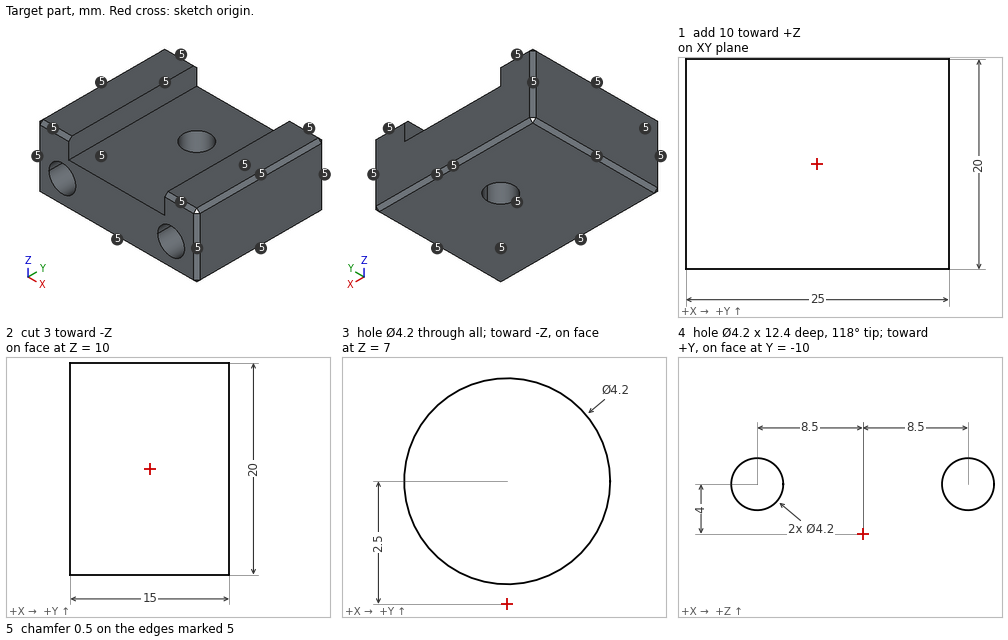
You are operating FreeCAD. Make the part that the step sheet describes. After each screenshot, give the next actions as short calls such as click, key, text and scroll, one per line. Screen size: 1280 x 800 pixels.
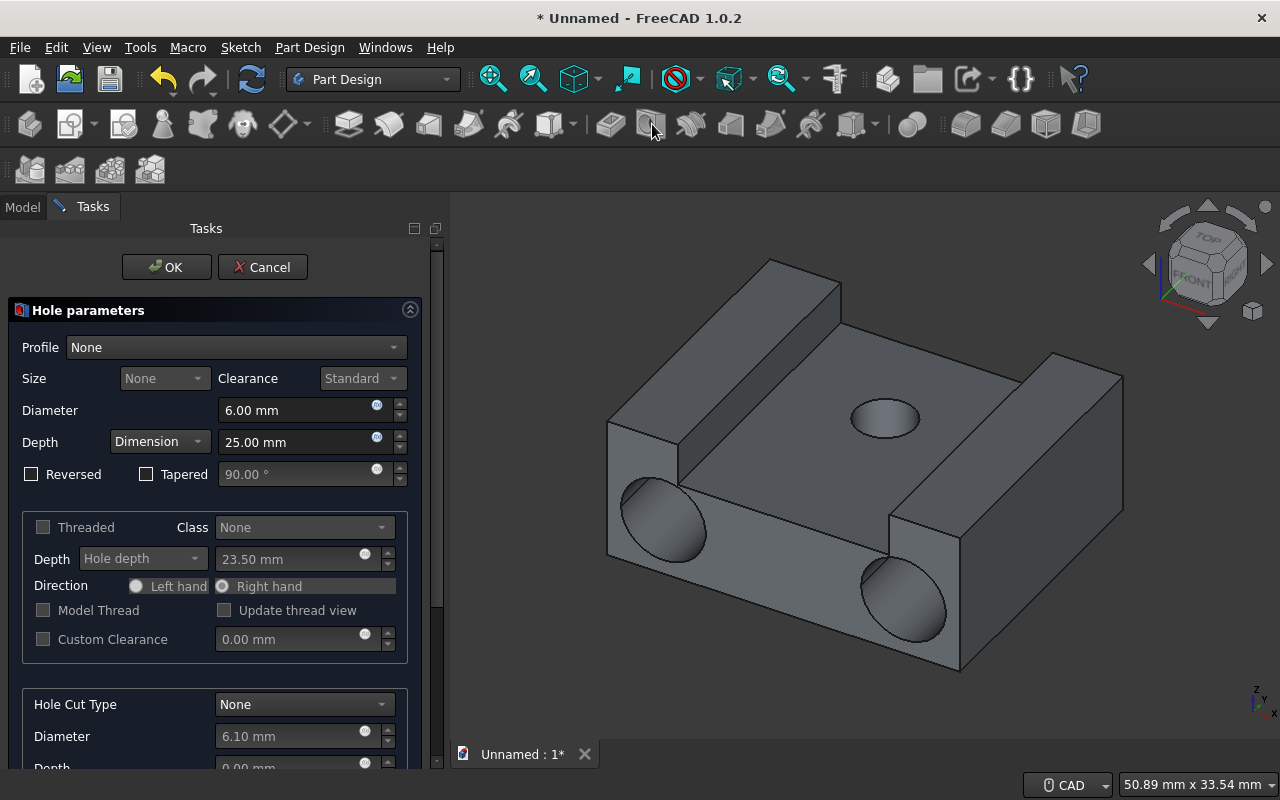
triple_click(305, 410)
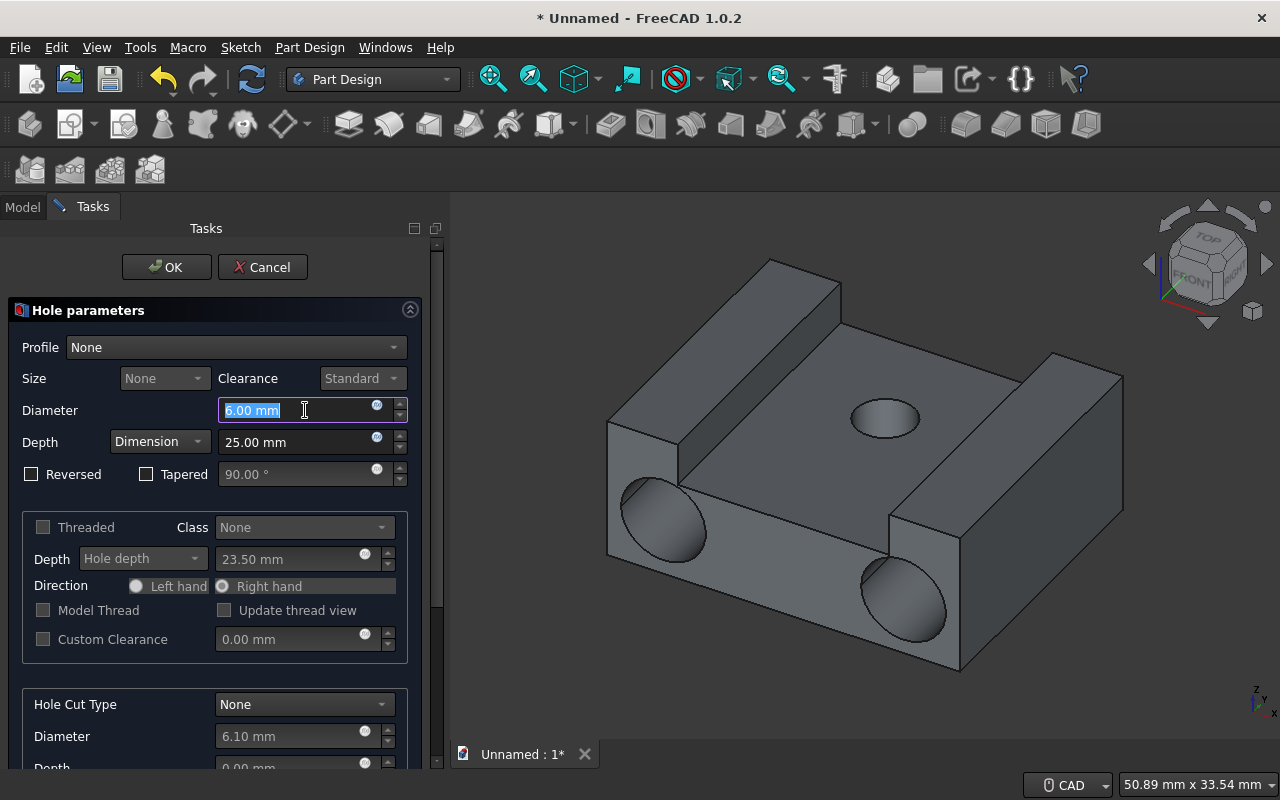
text(4.2)
key(Tab)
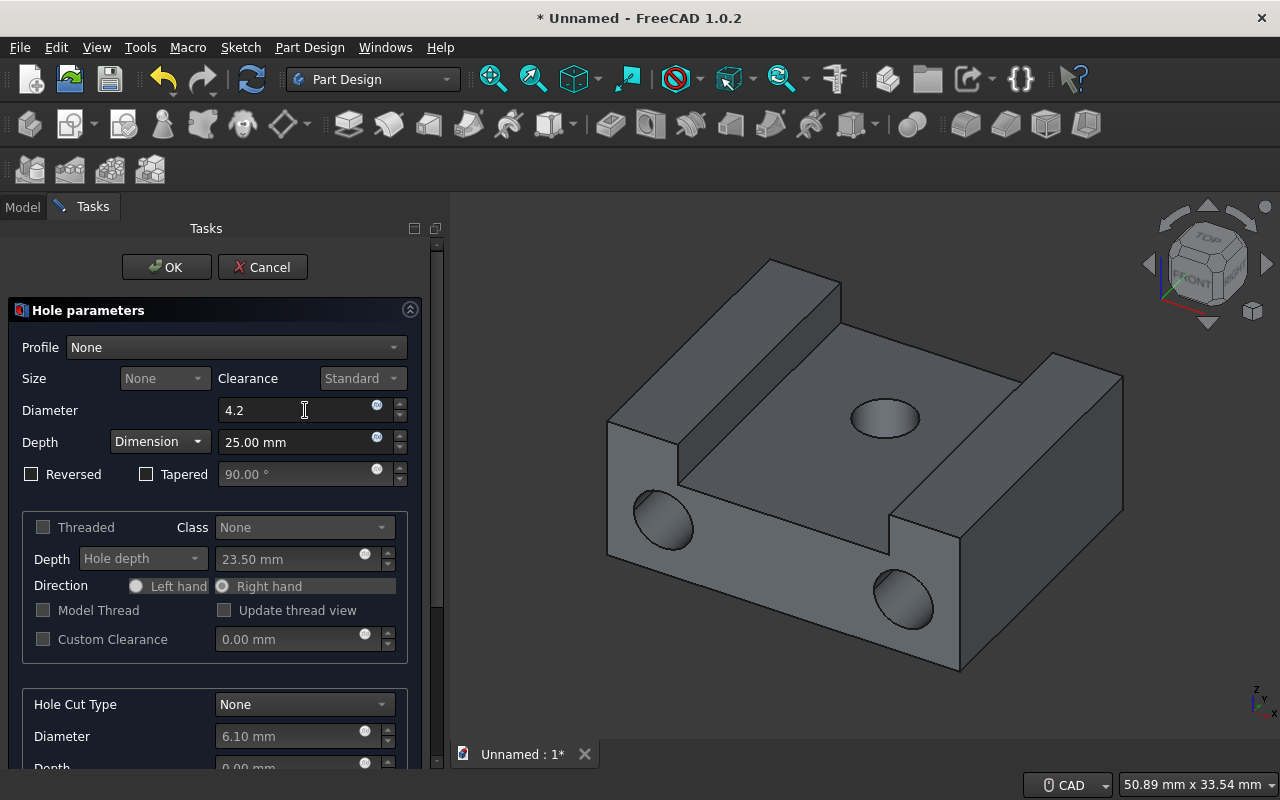
triple_click(305, 442)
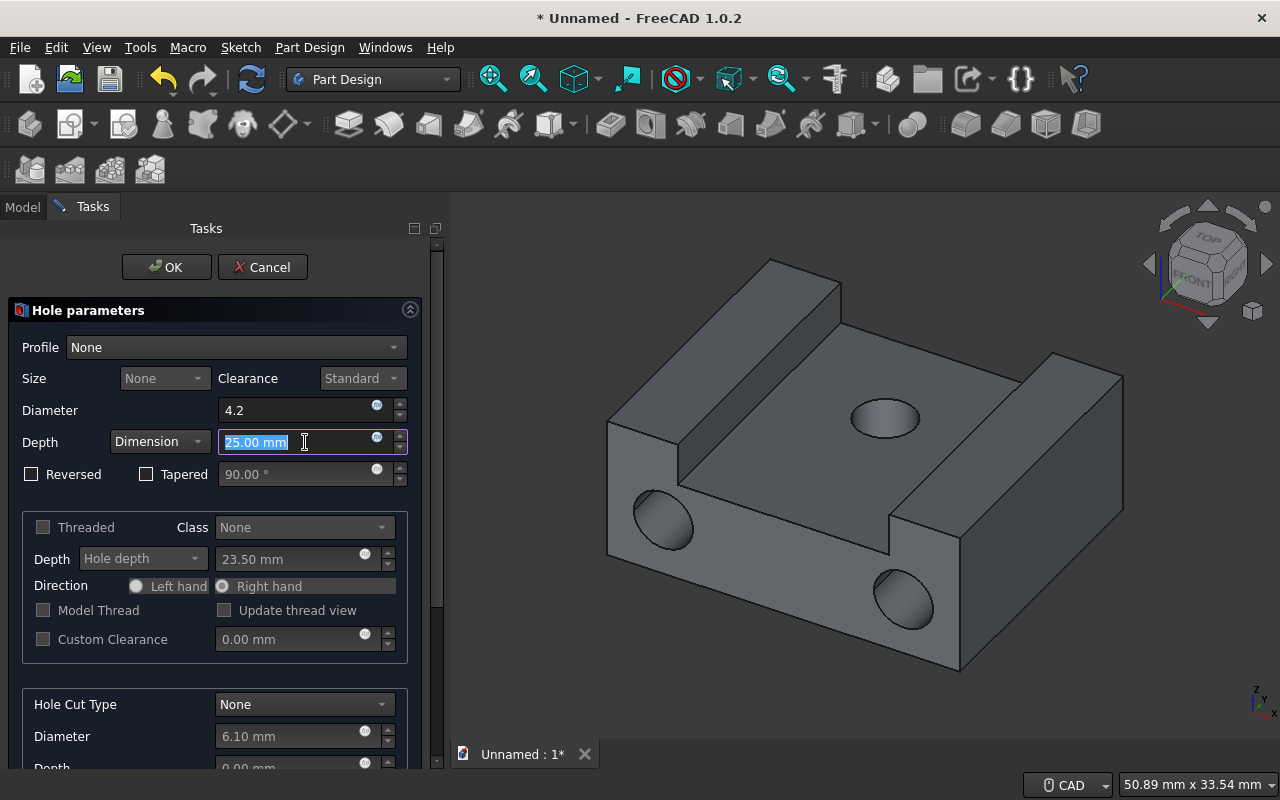
text(12.4)
key(Tab)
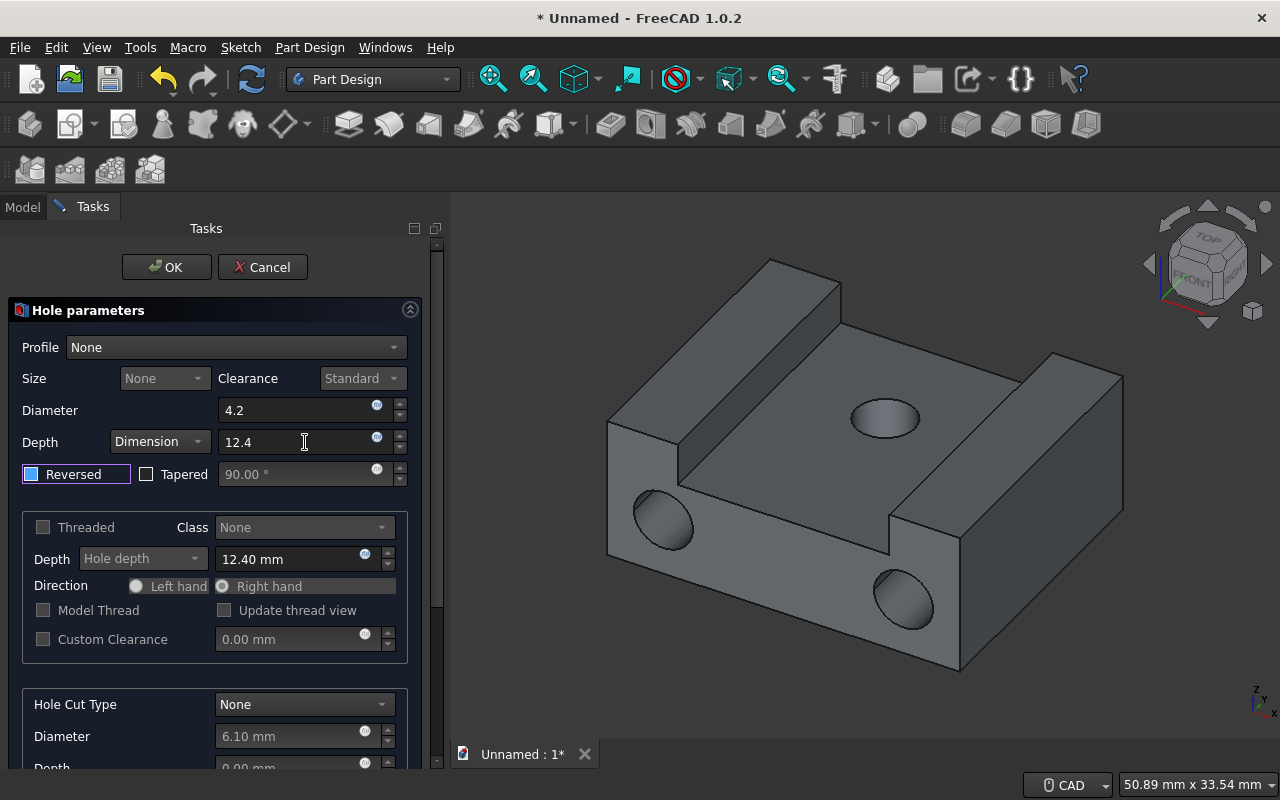
click(167, 267)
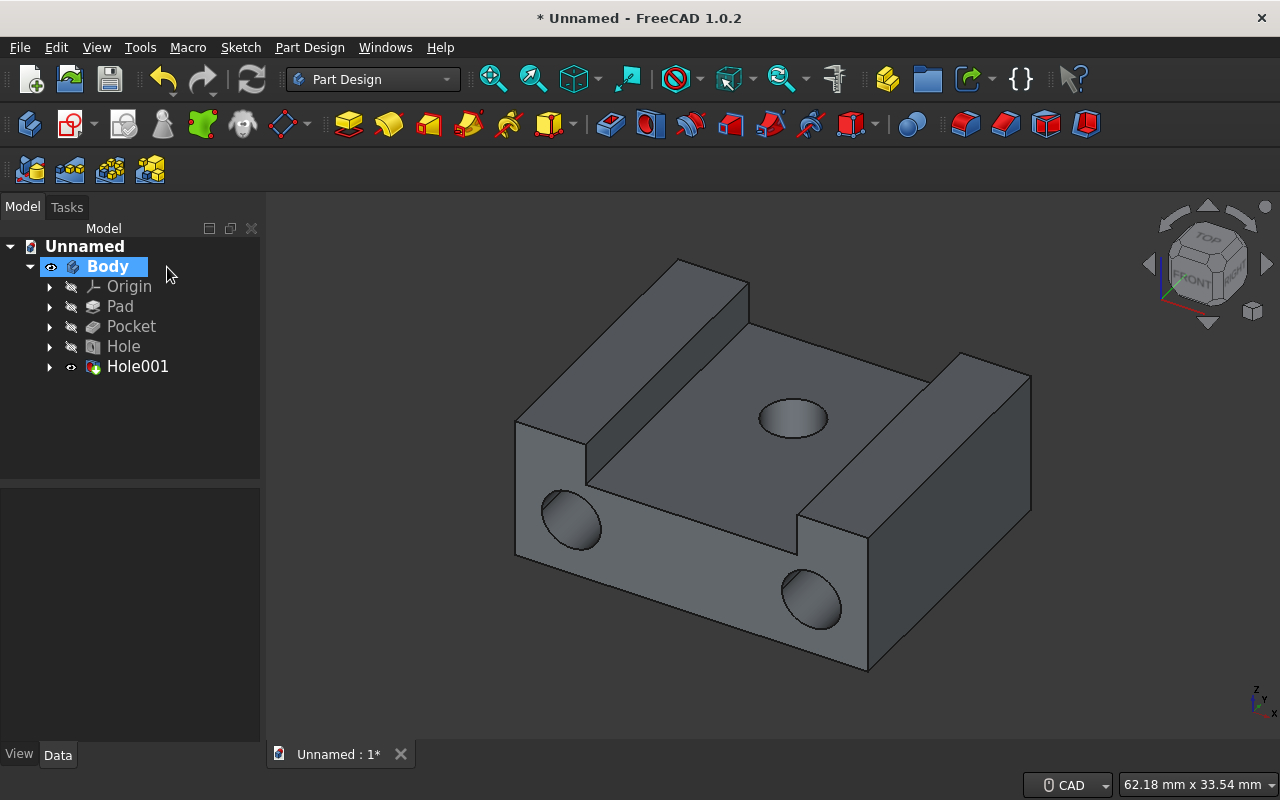
click(973, 500)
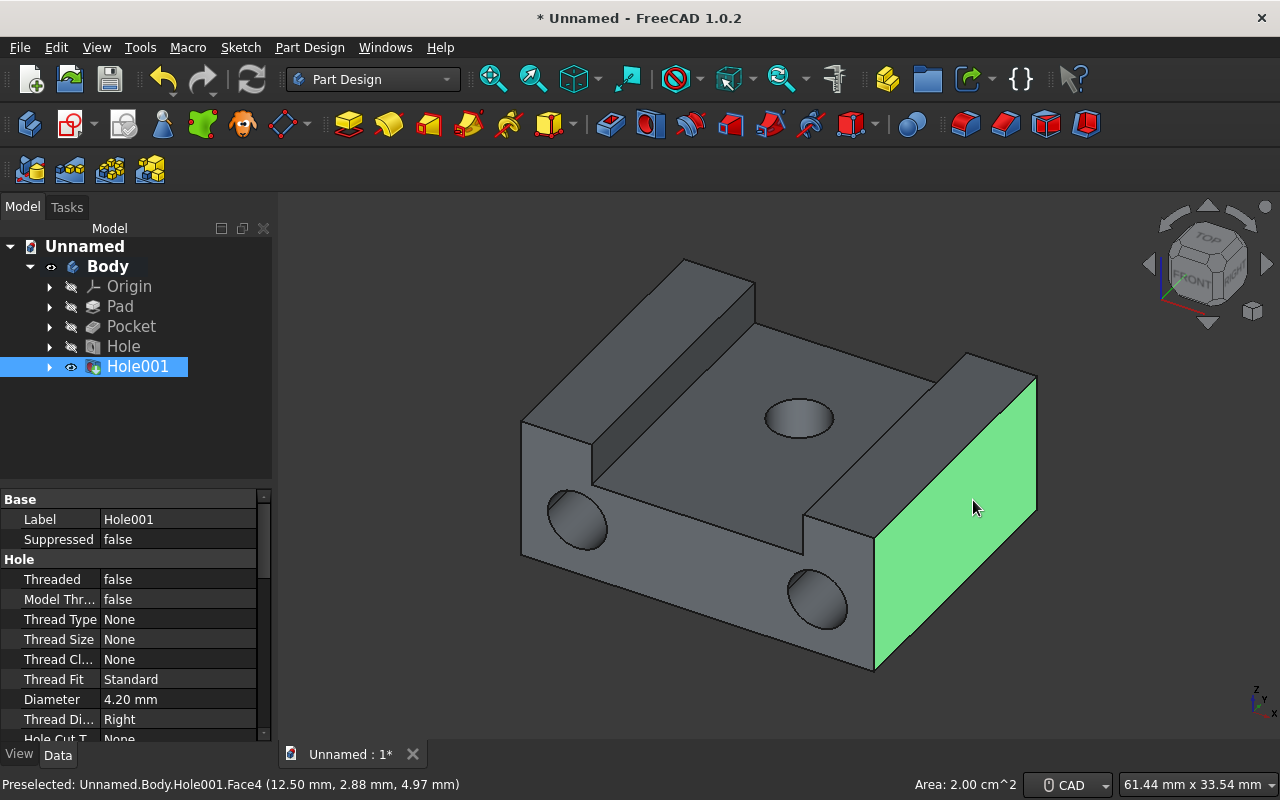
click(556, 432, ctrl)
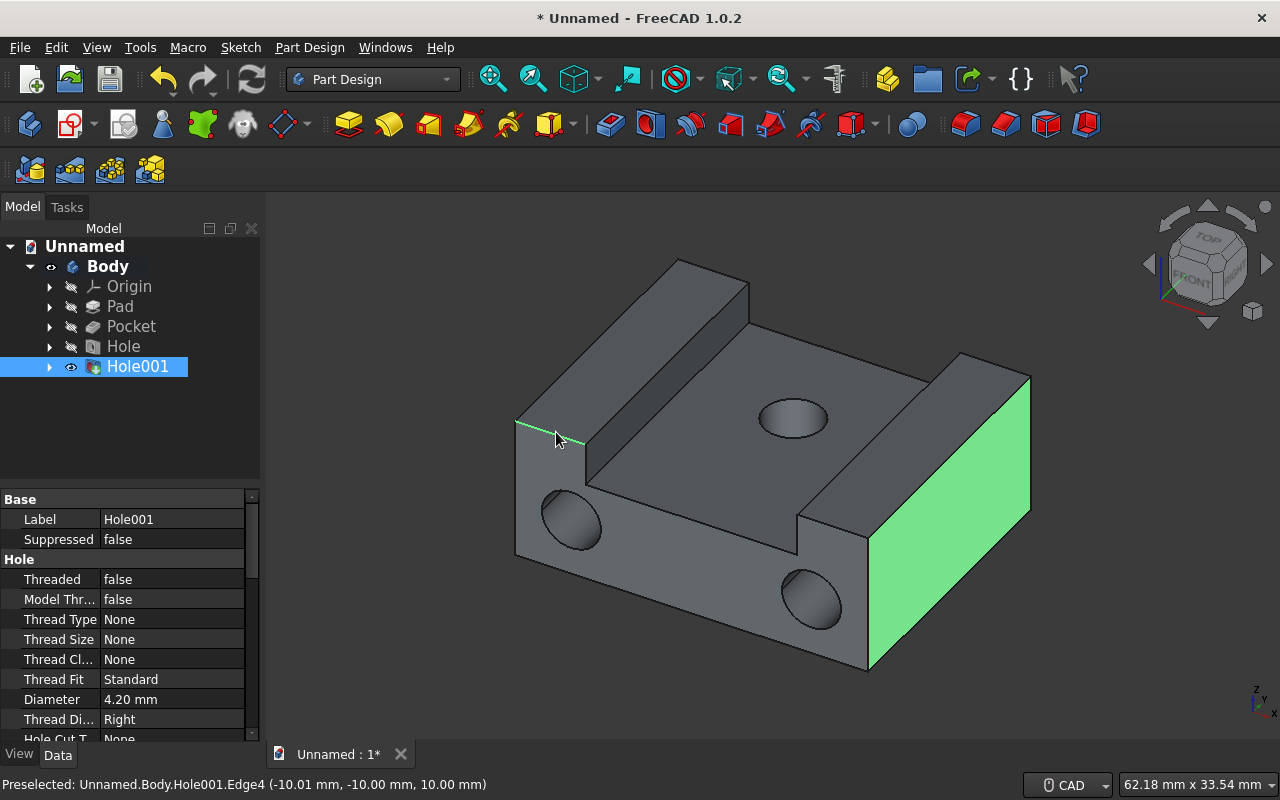
click(833, 525, ctrl)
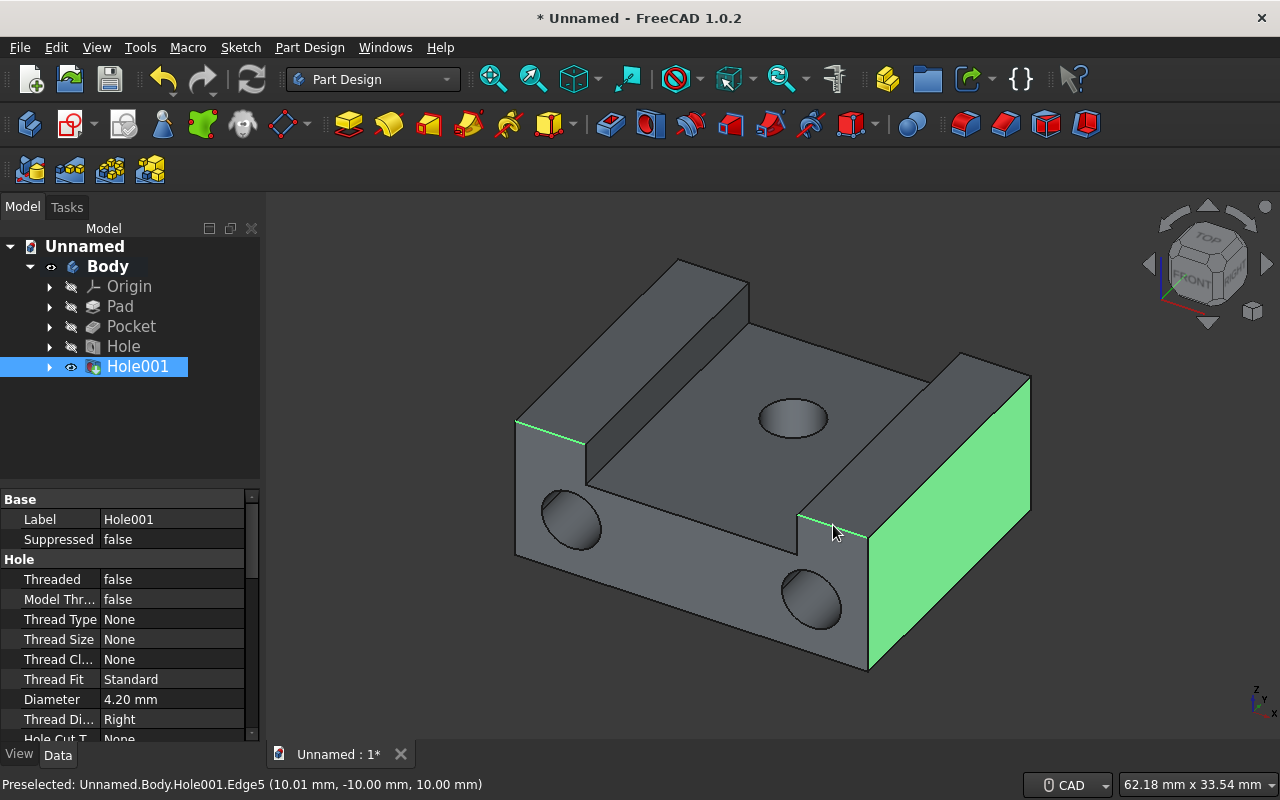
key(0)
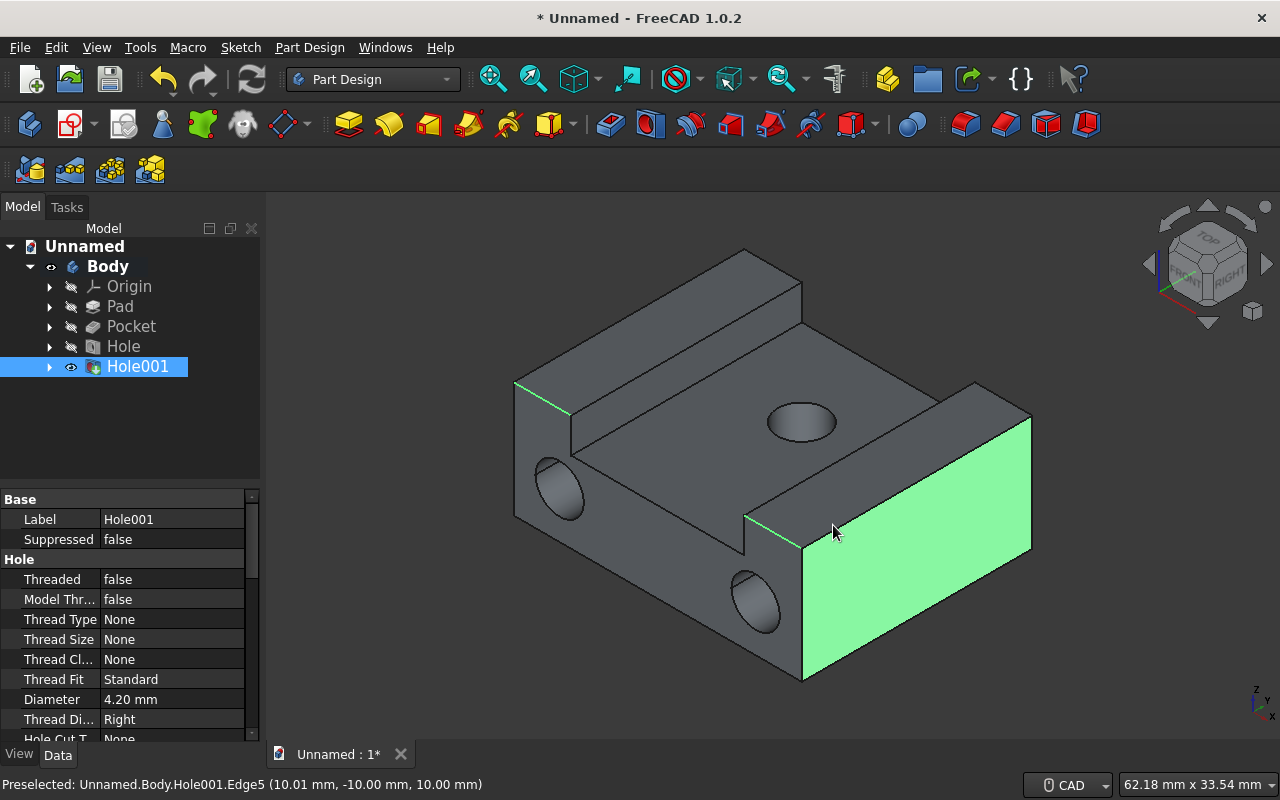
key(2)